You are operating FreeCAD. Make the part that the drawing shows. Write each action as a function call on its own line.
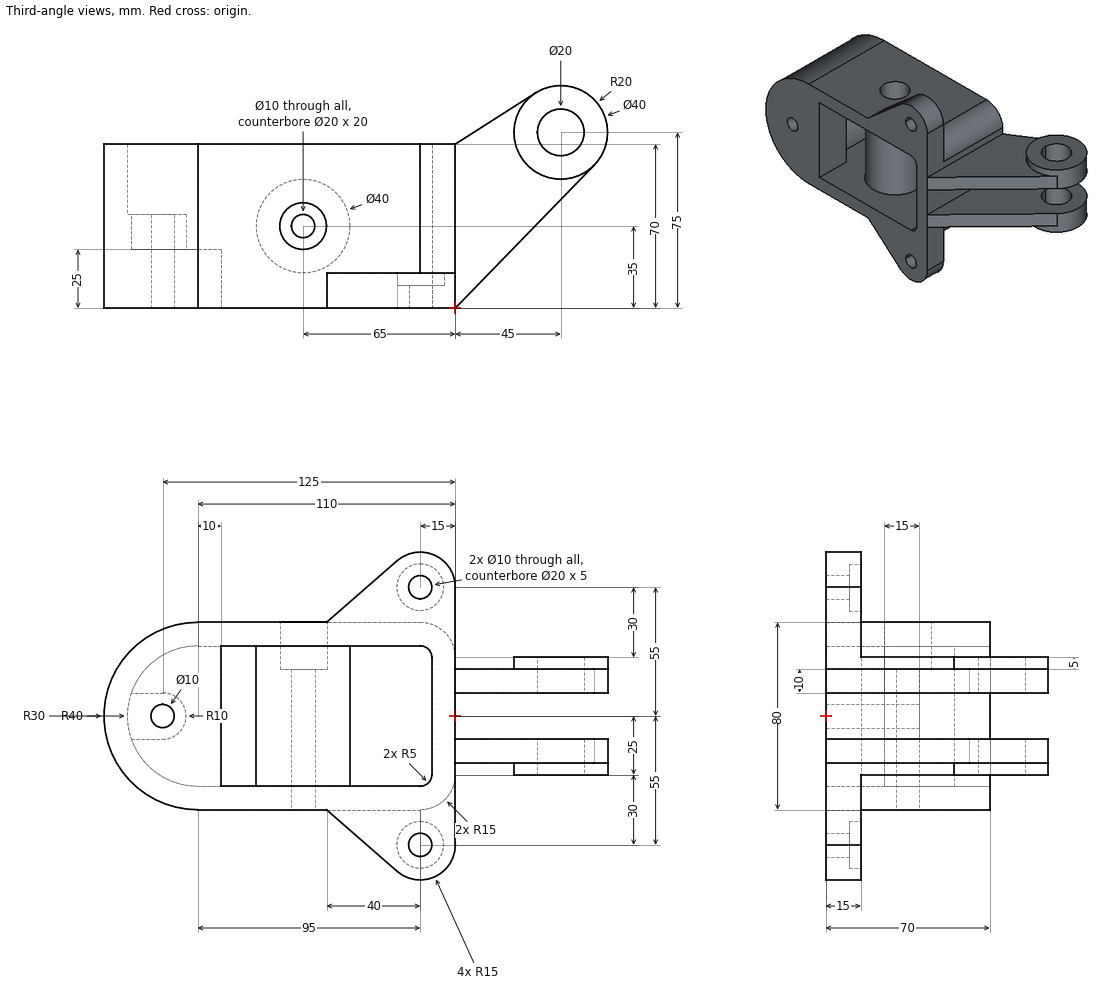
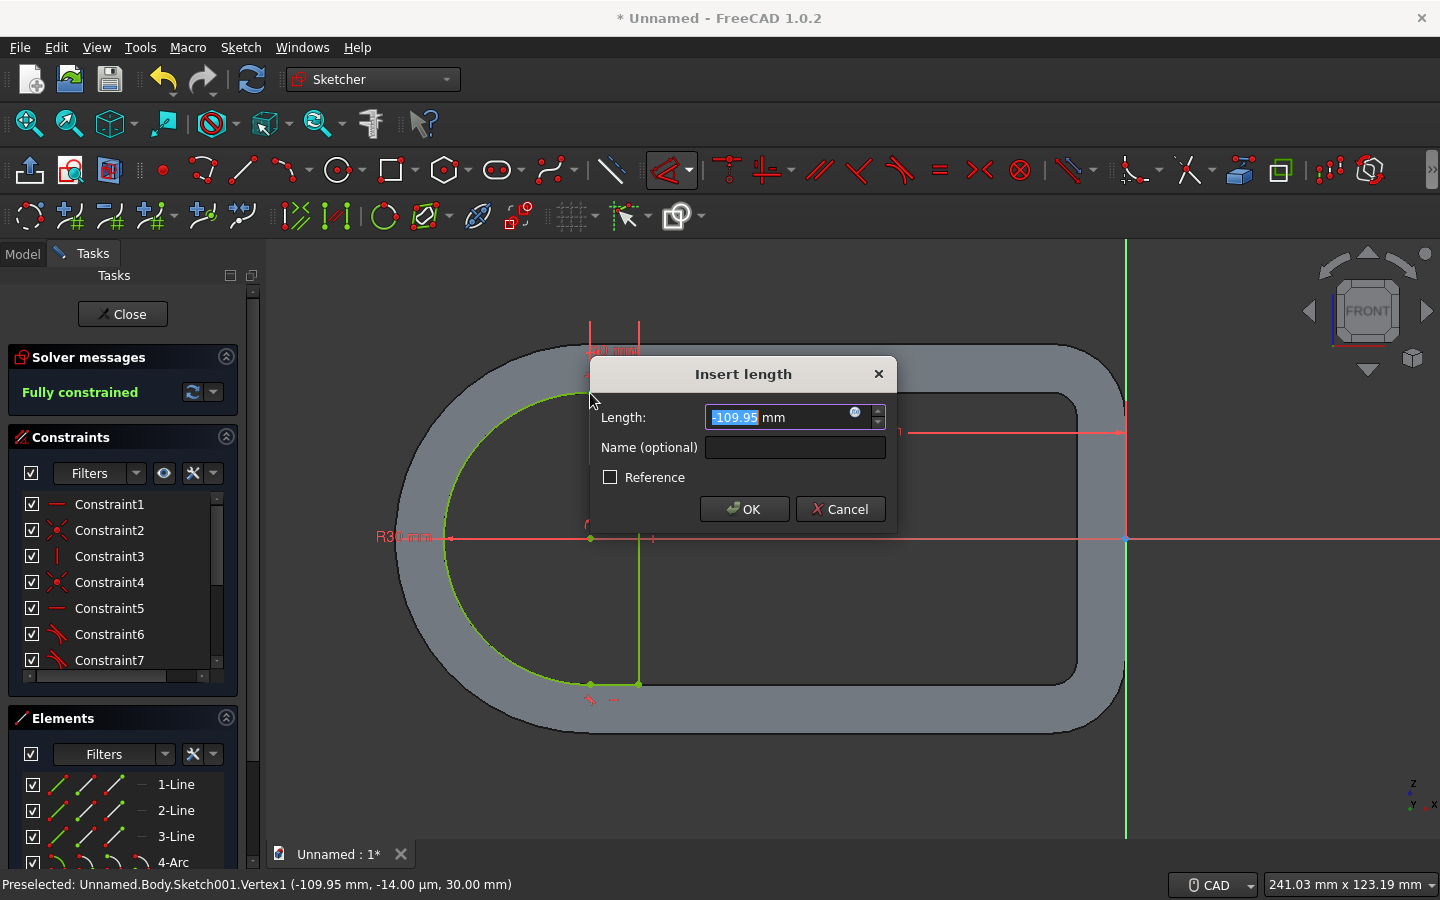
text(-110)
key(Return)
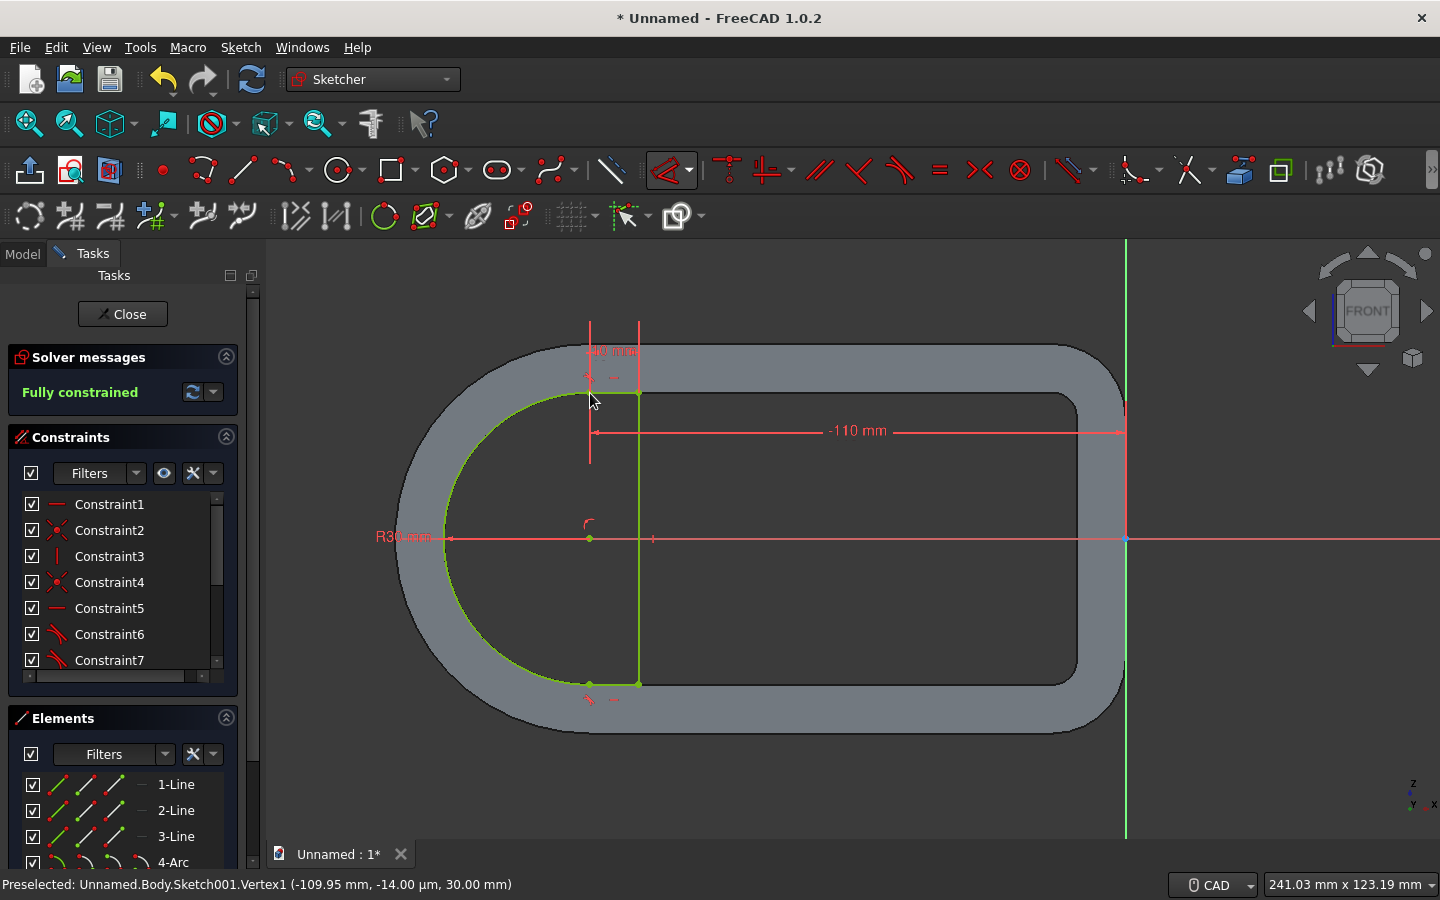
click(123, 314)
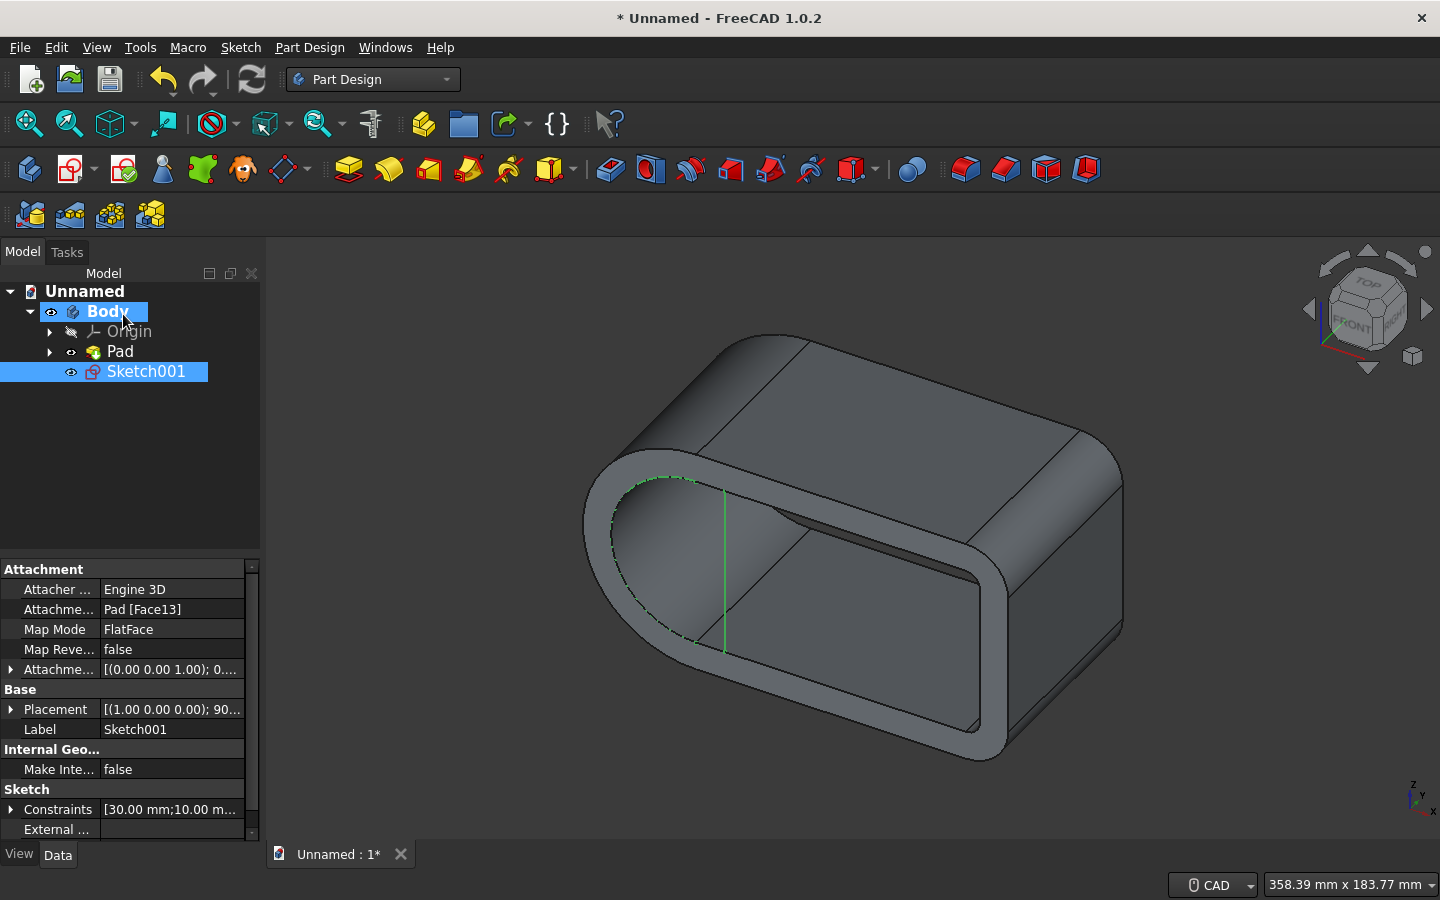
click(350, 170)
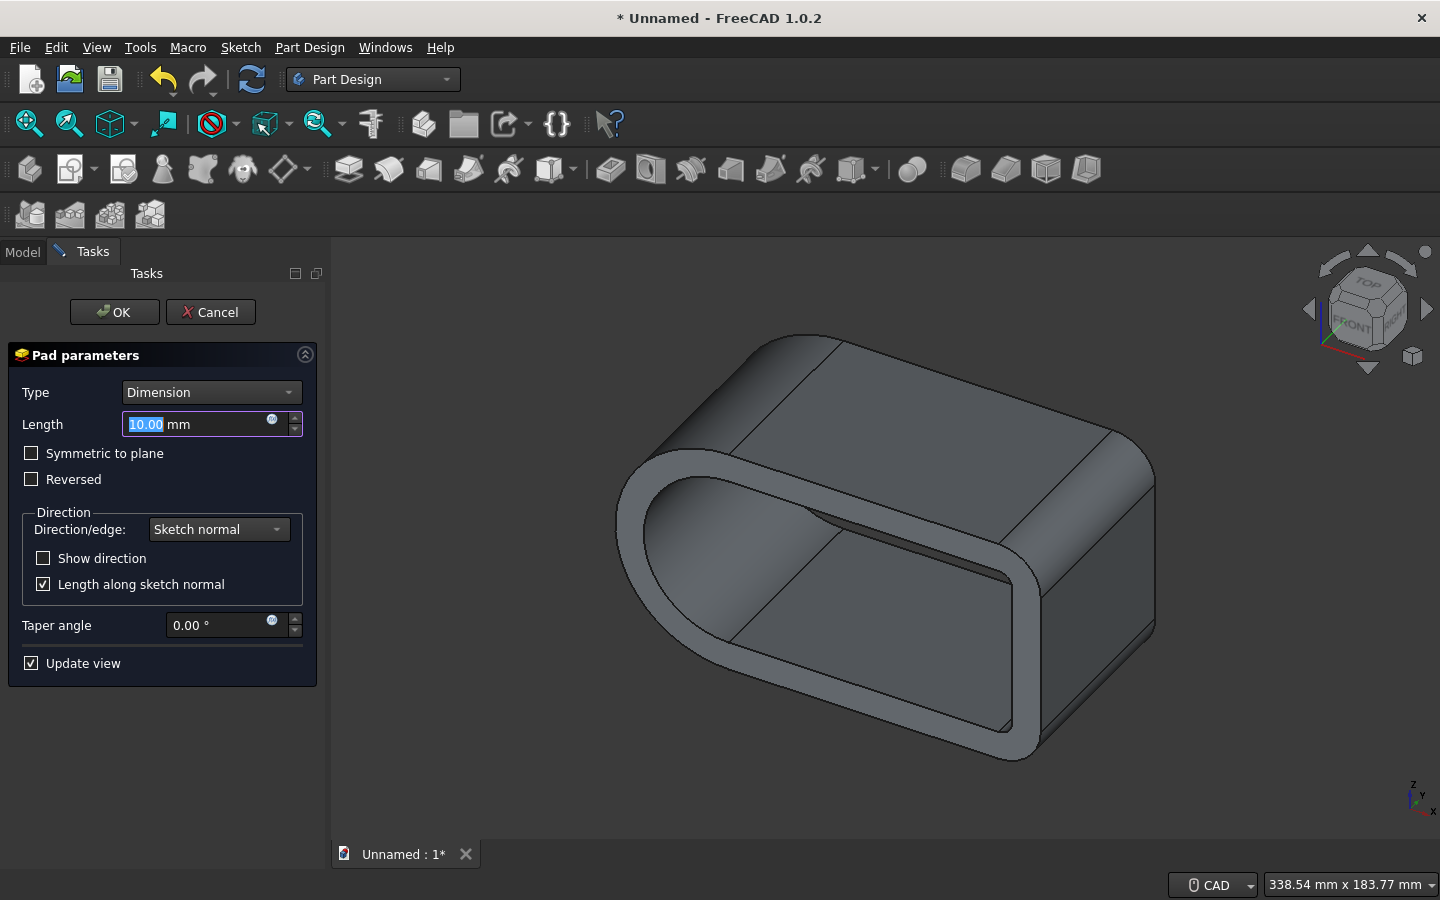
text(25)
key(Tab)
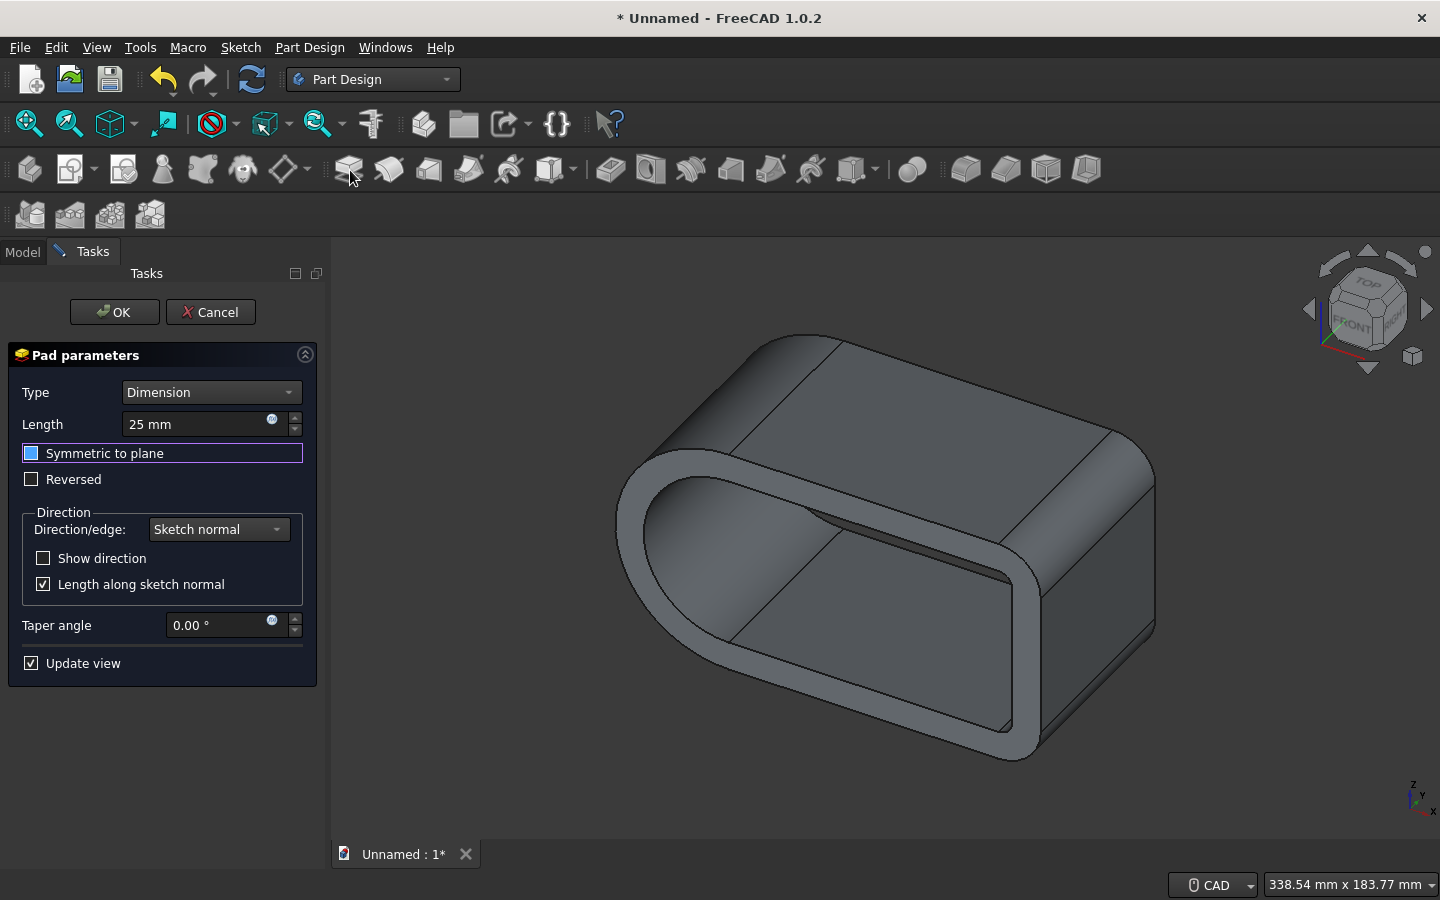
click(30, 479)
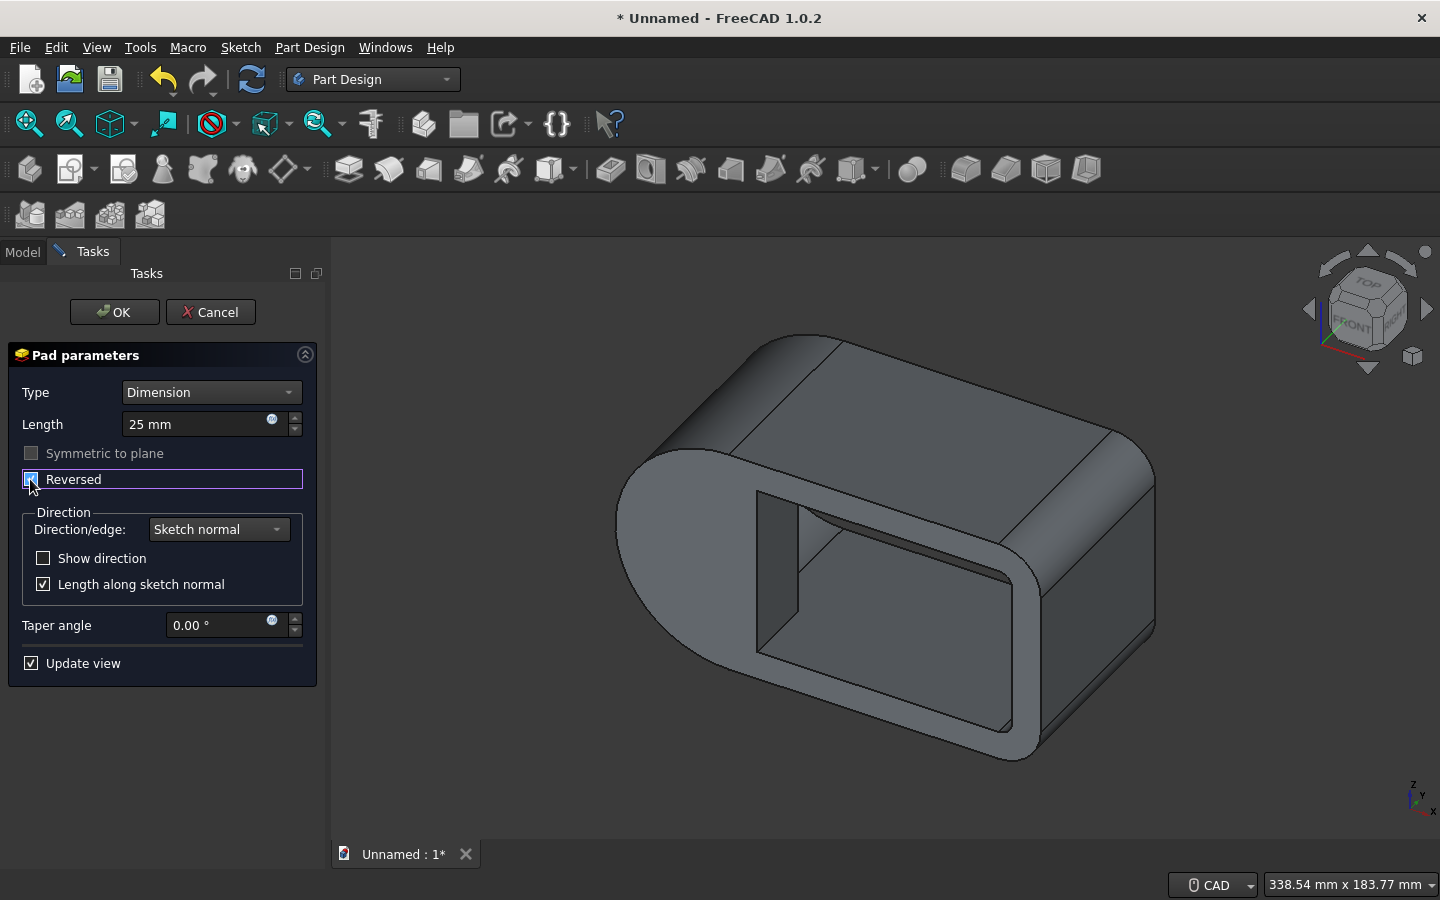
click(115, 312)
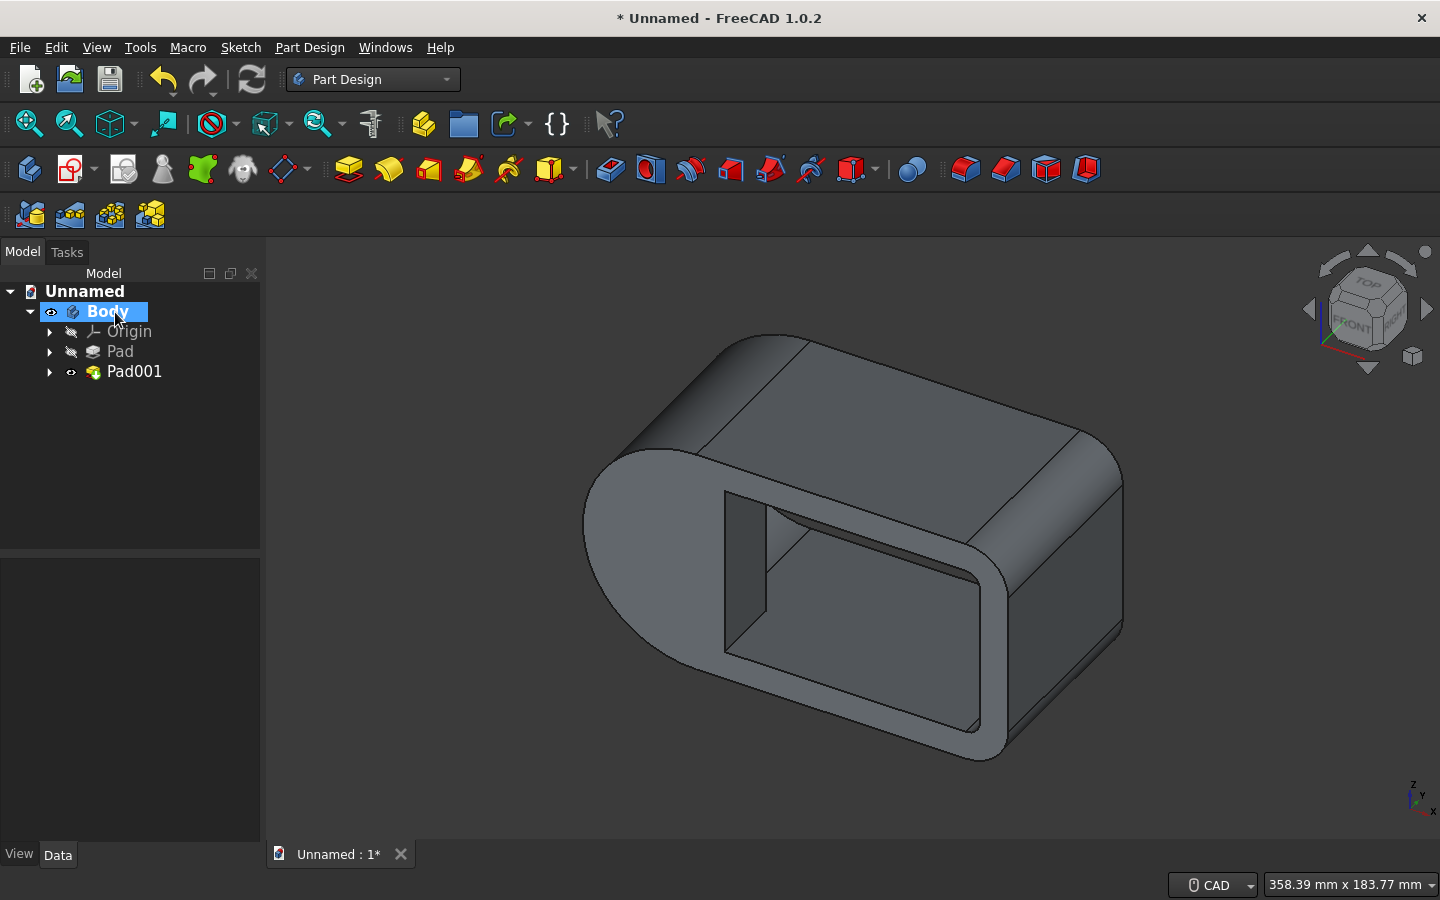
key(4)